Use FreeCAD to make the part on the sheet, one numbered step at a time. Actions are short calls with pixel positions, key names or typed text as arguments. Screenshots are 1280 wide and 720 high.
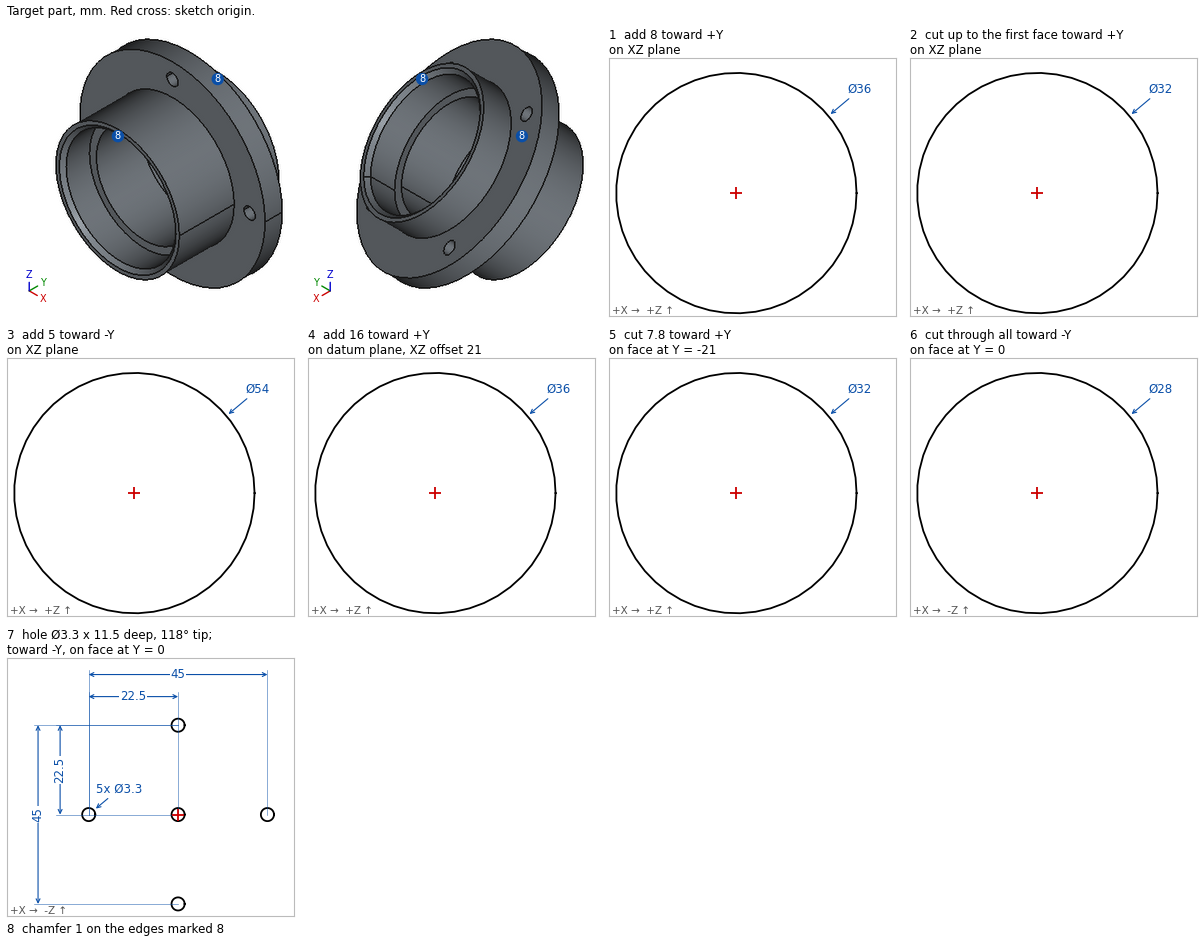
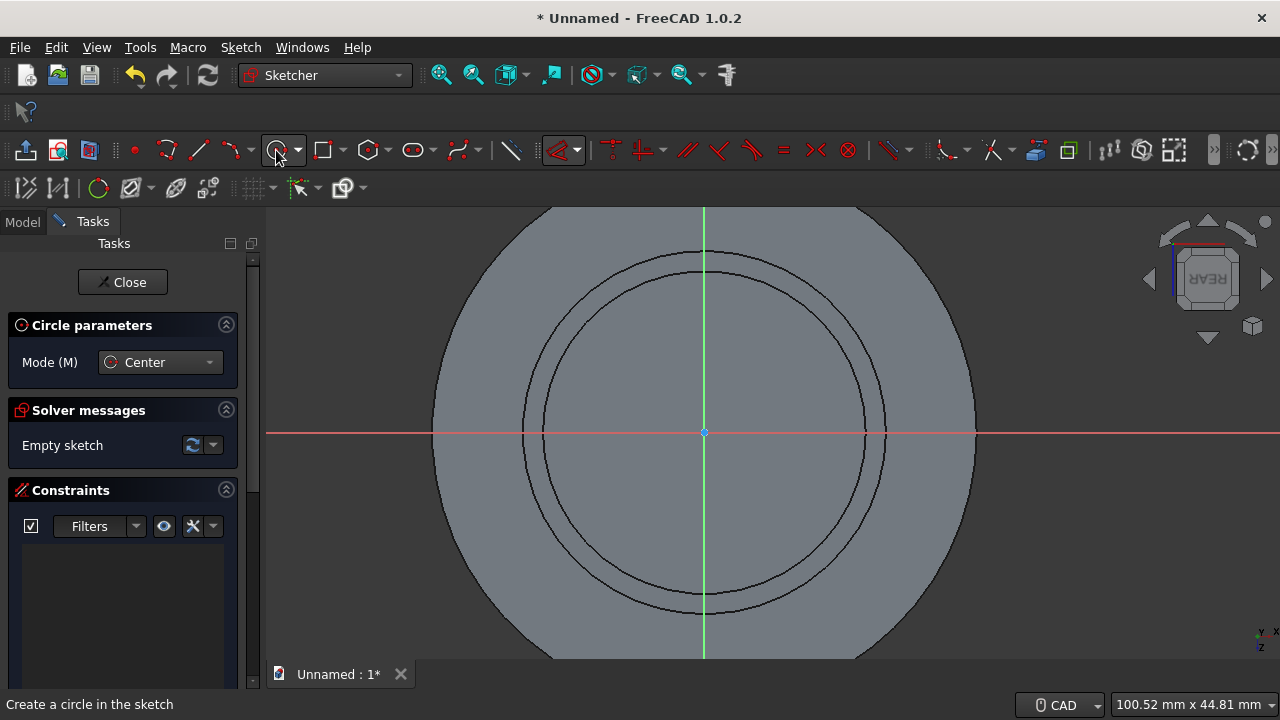
click(704, 433)
click(804, 333)
key(Escape)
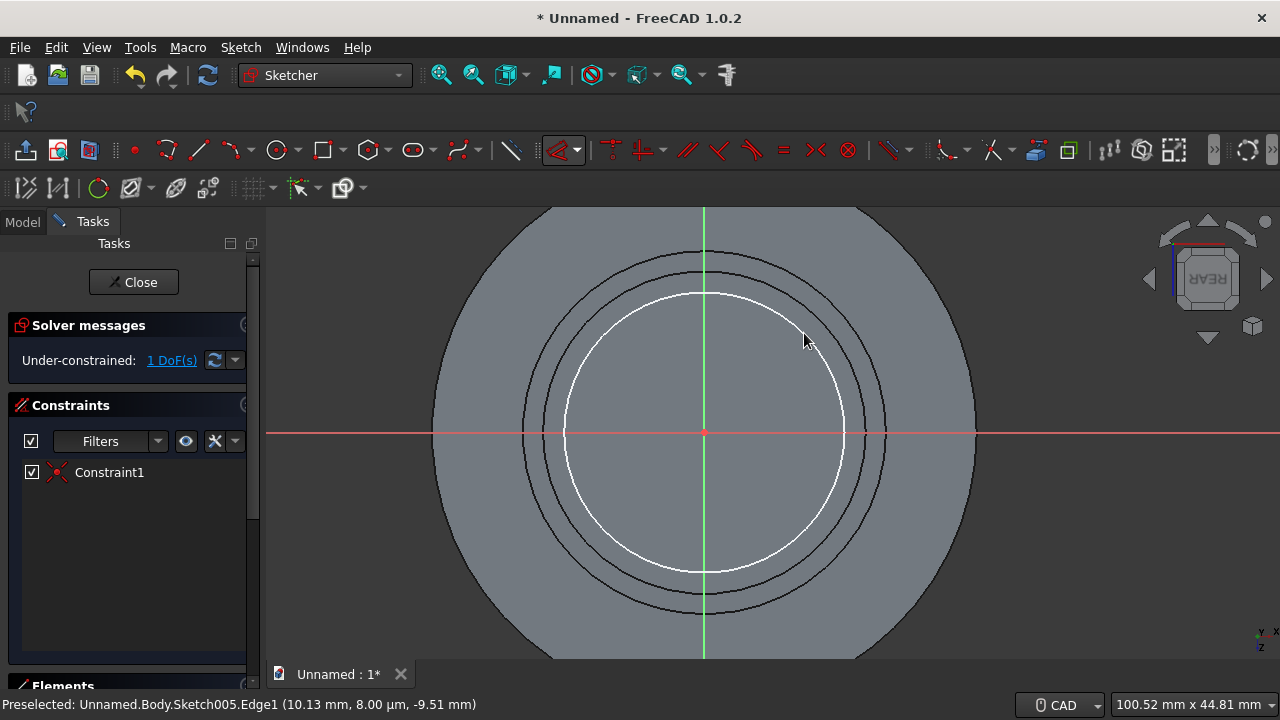
click(803, 333)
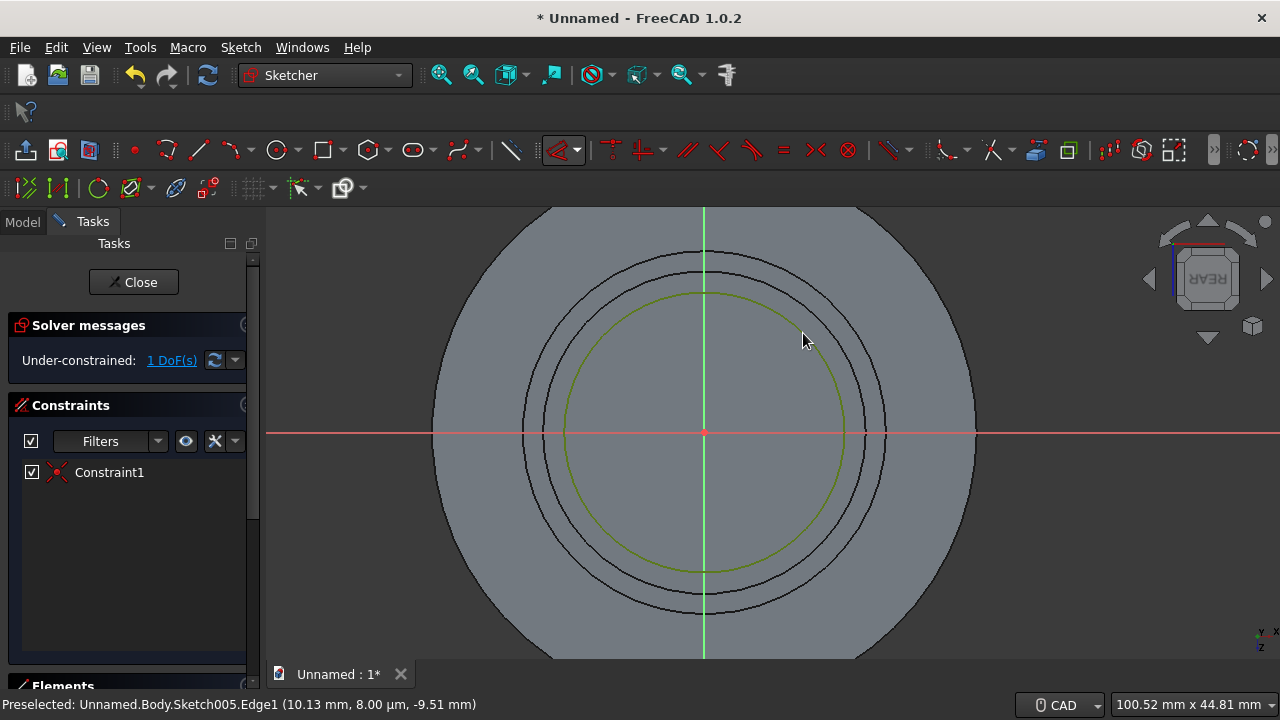
click(580, 150)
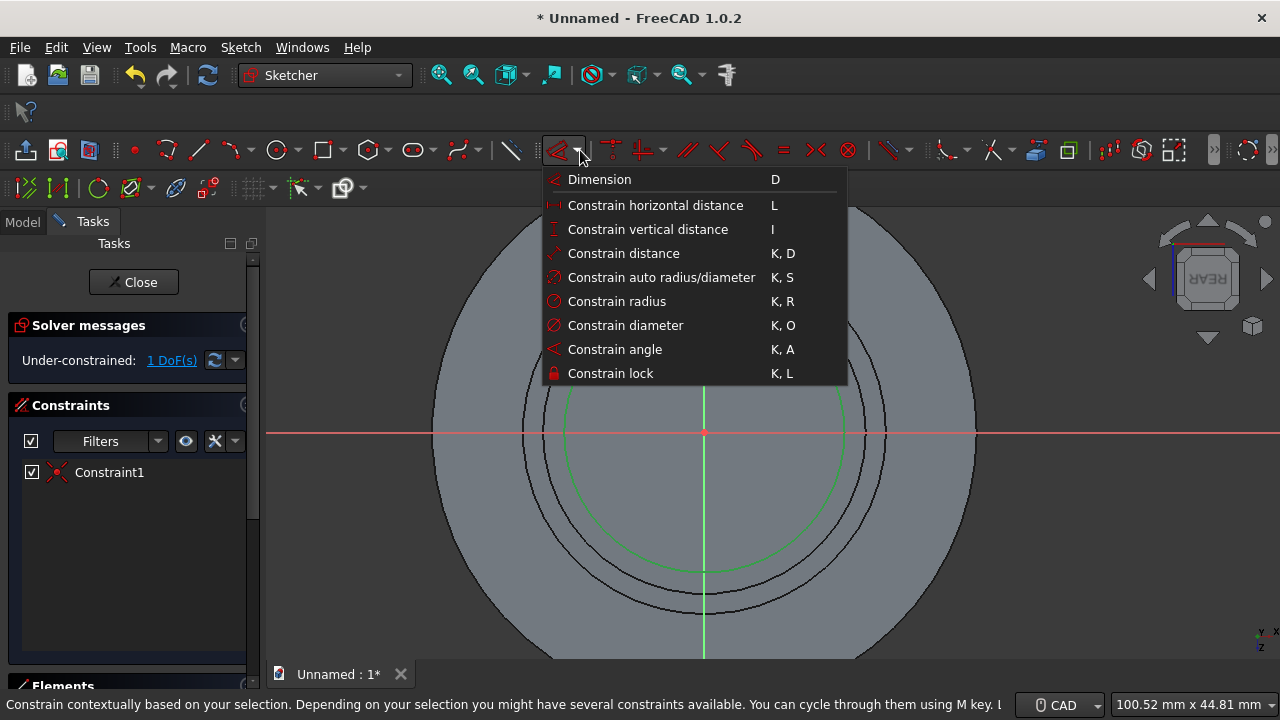
click(695, 325)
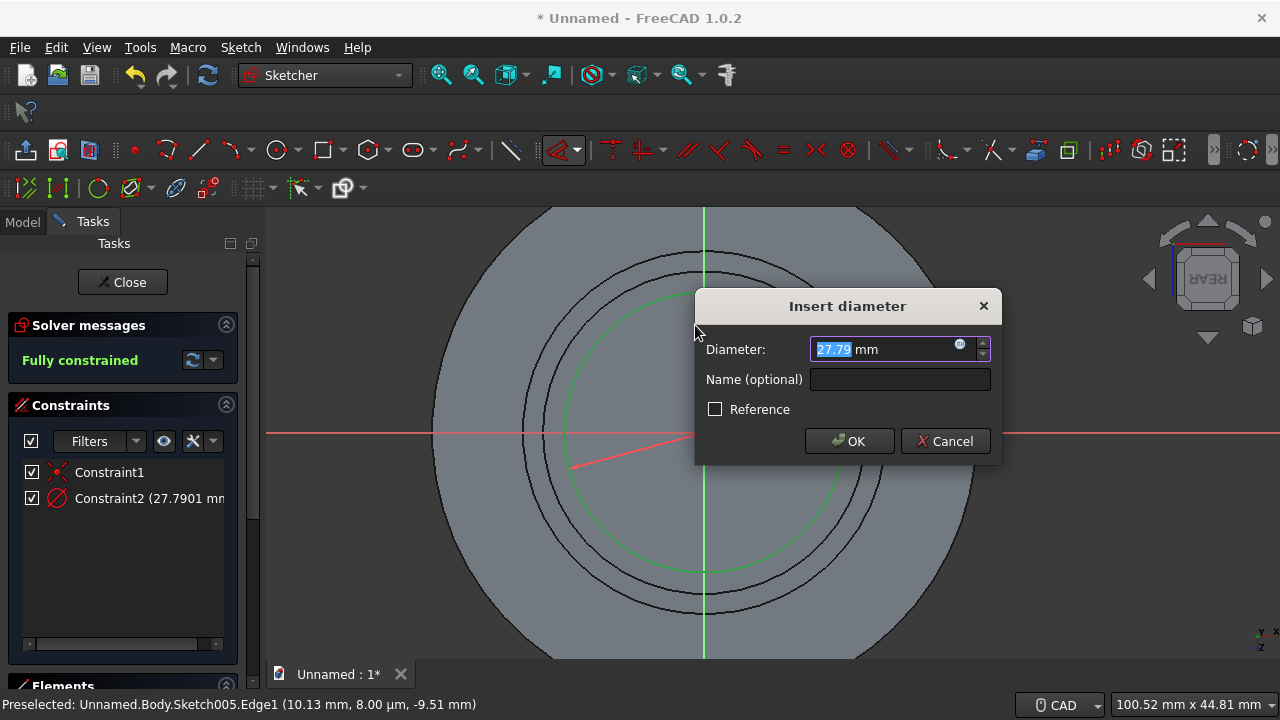
text(28)
key(Return)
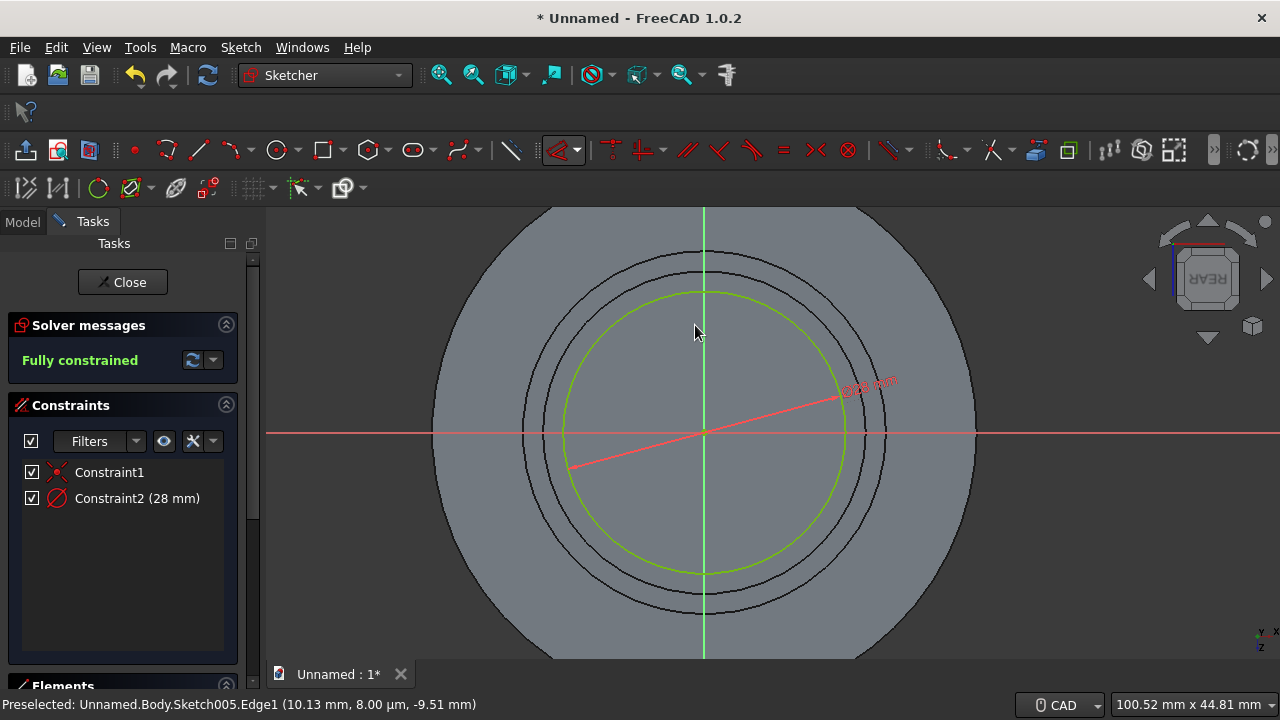
click(123, 282)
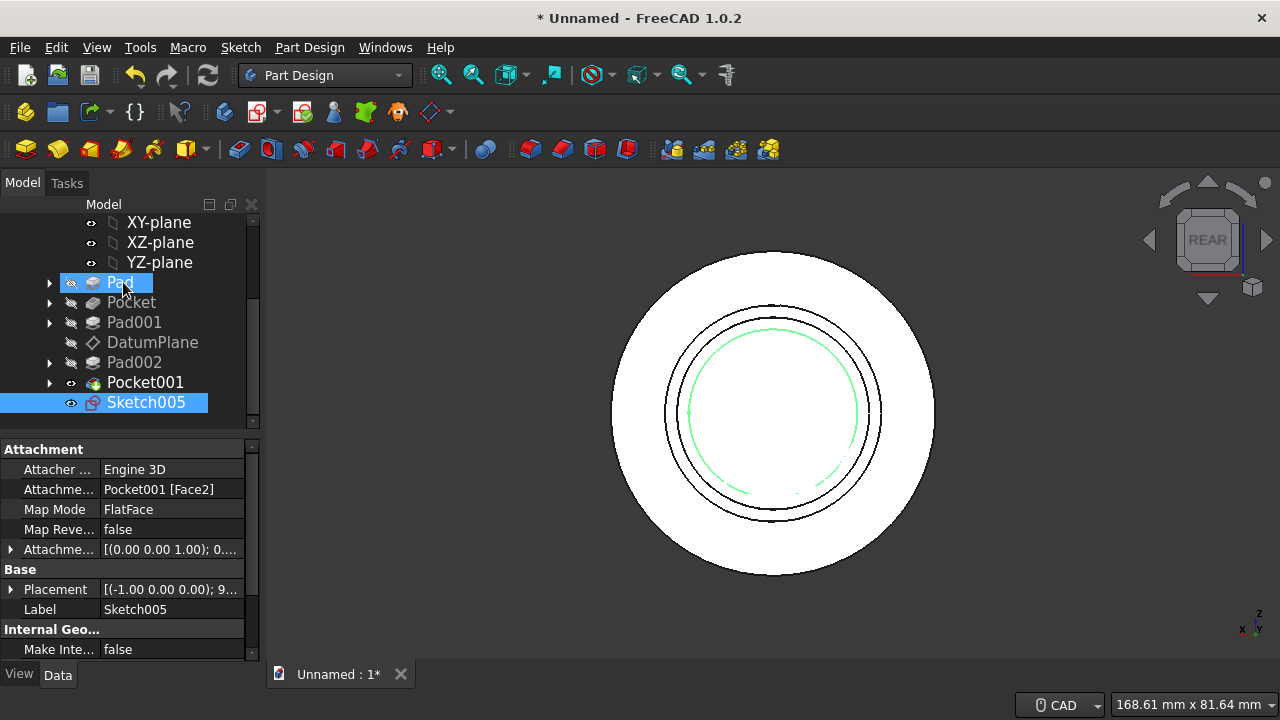
click(240, 150)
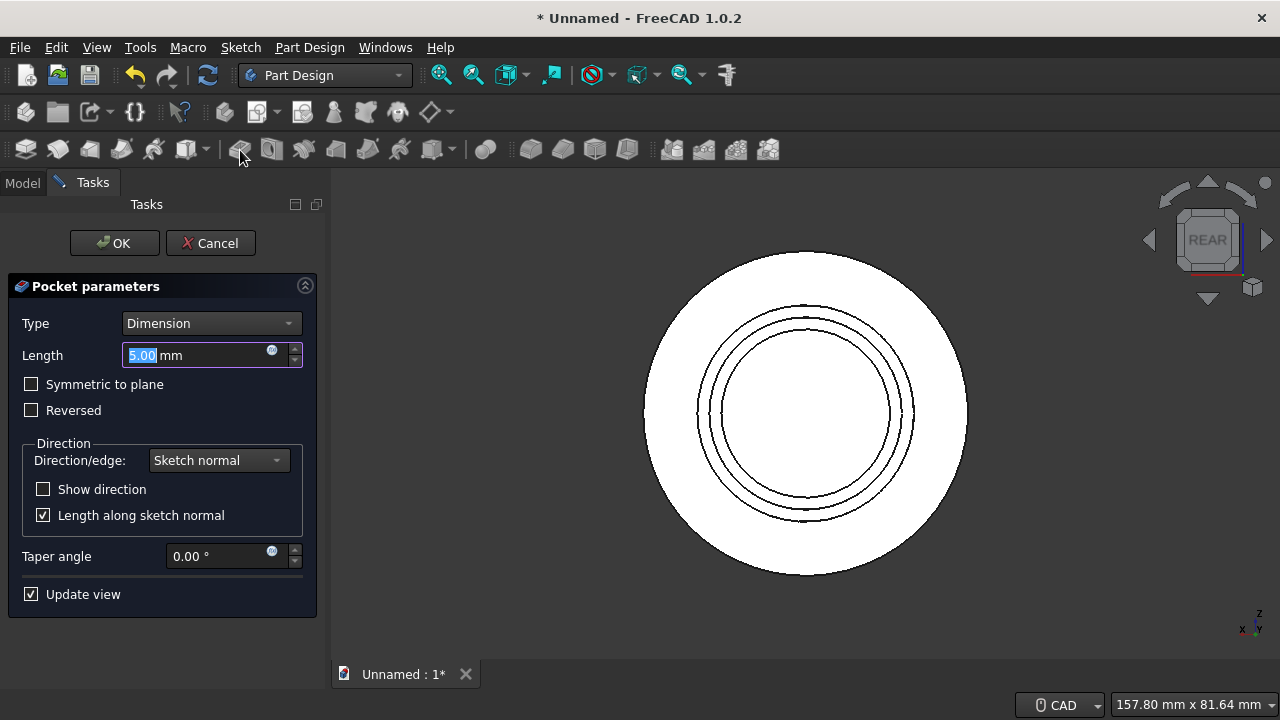
click(212, 324)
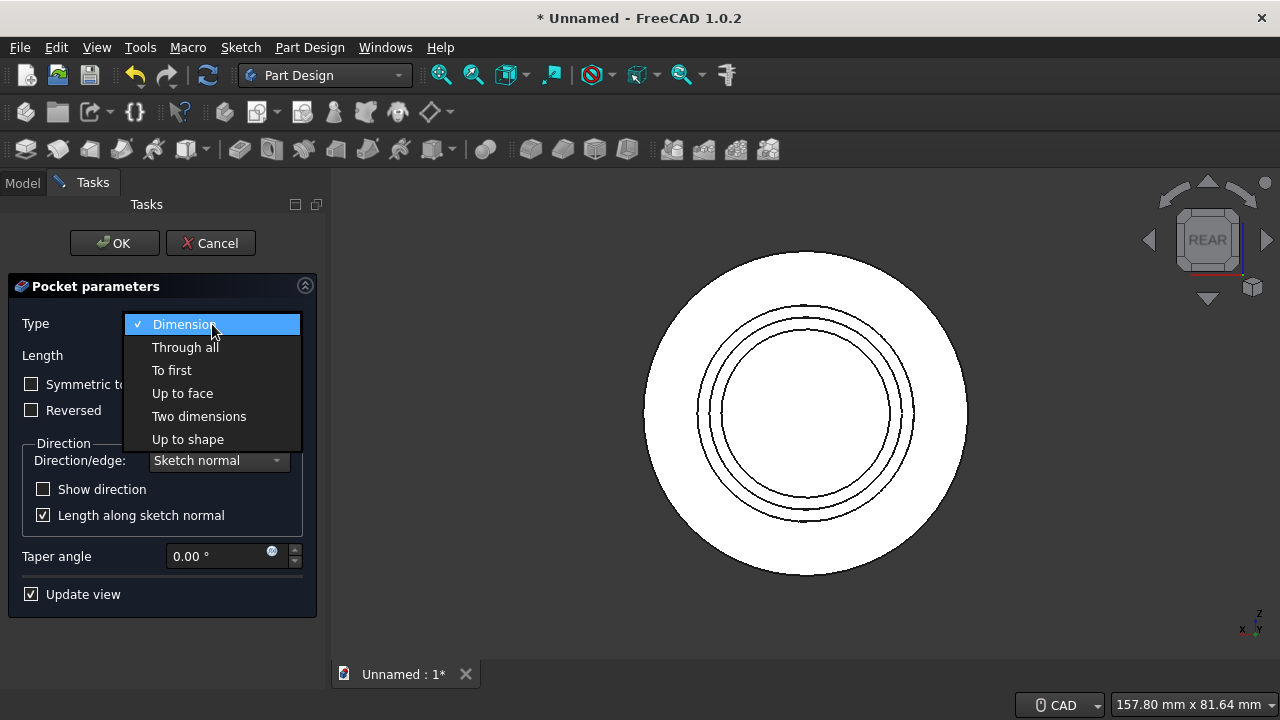
click(212, 348)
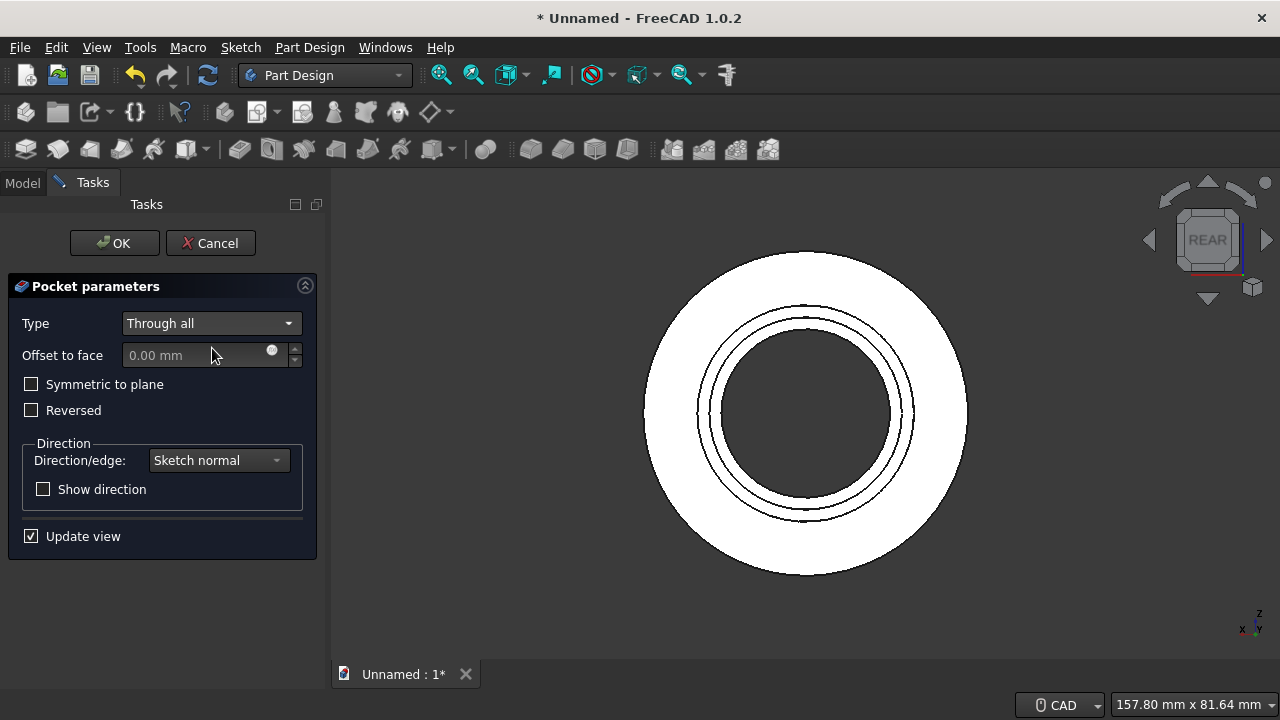
click(115, 243)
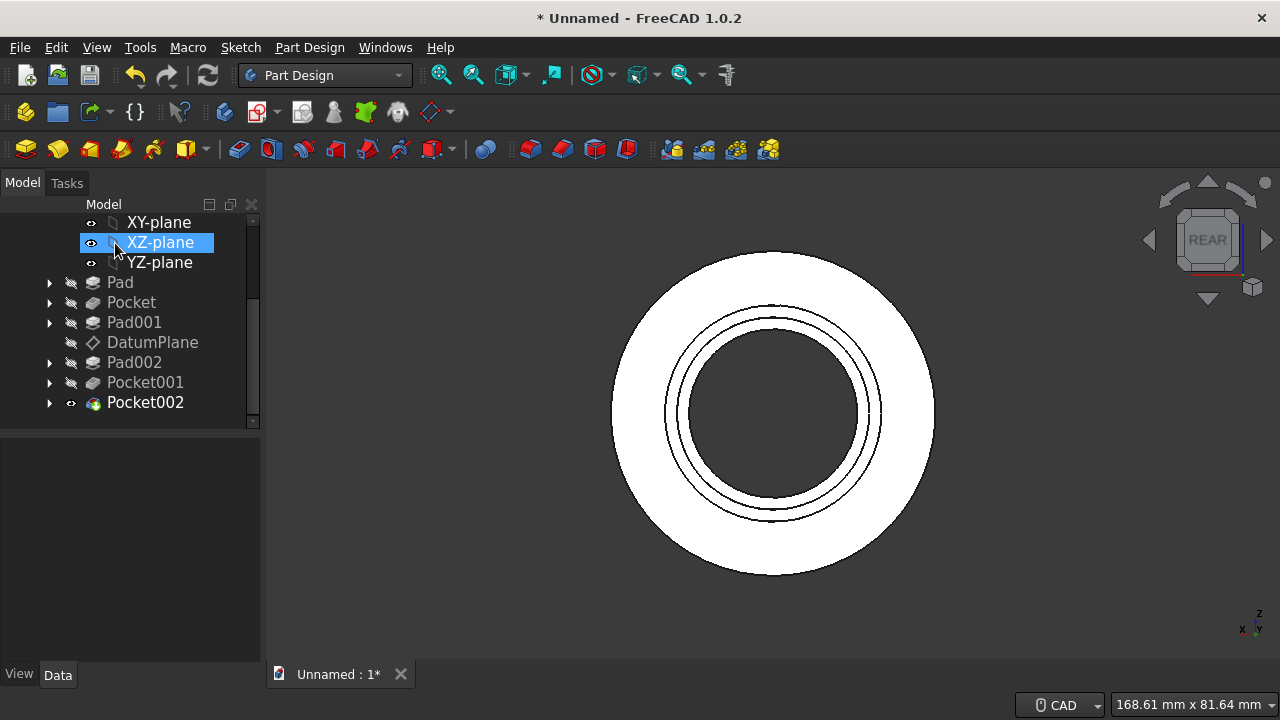
click(773, 552)